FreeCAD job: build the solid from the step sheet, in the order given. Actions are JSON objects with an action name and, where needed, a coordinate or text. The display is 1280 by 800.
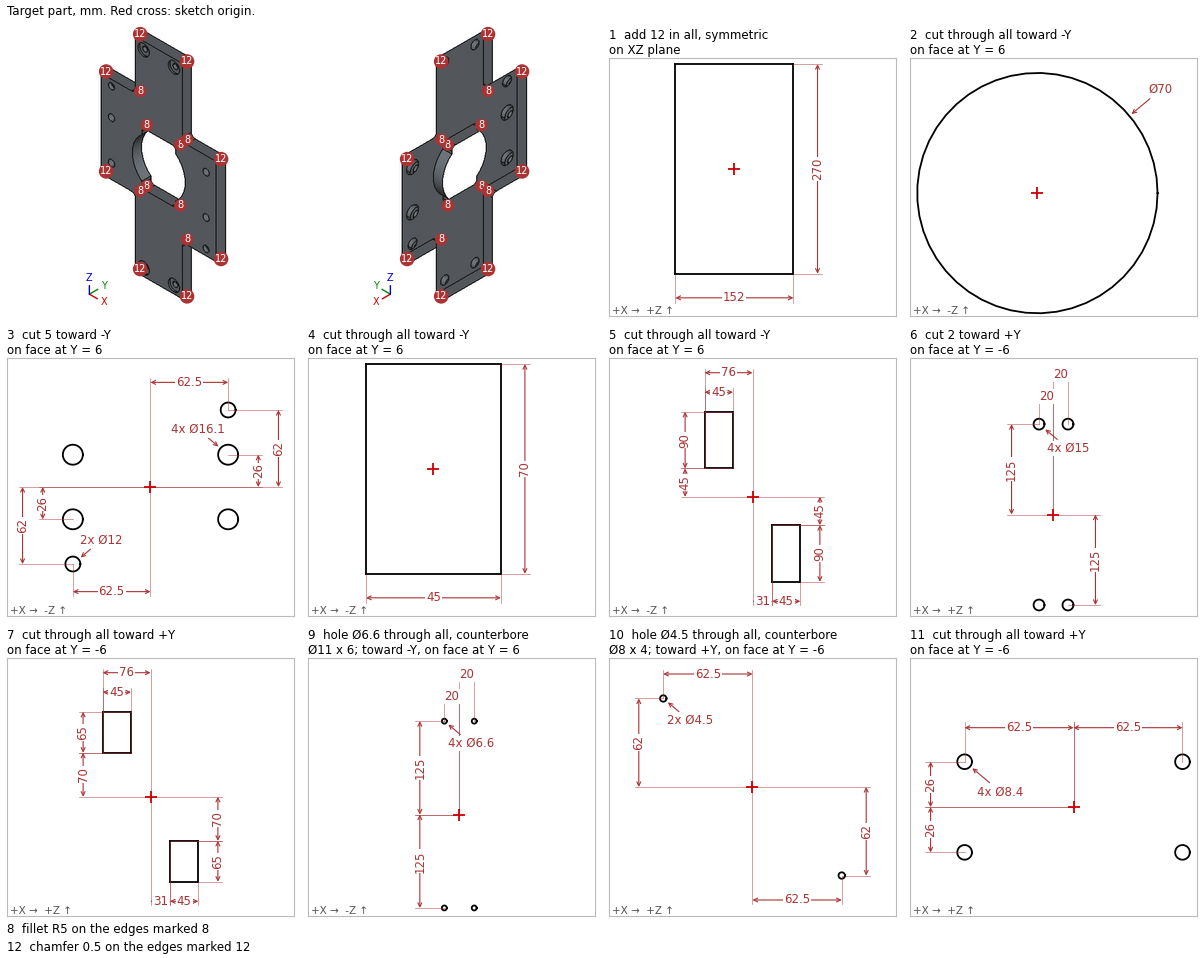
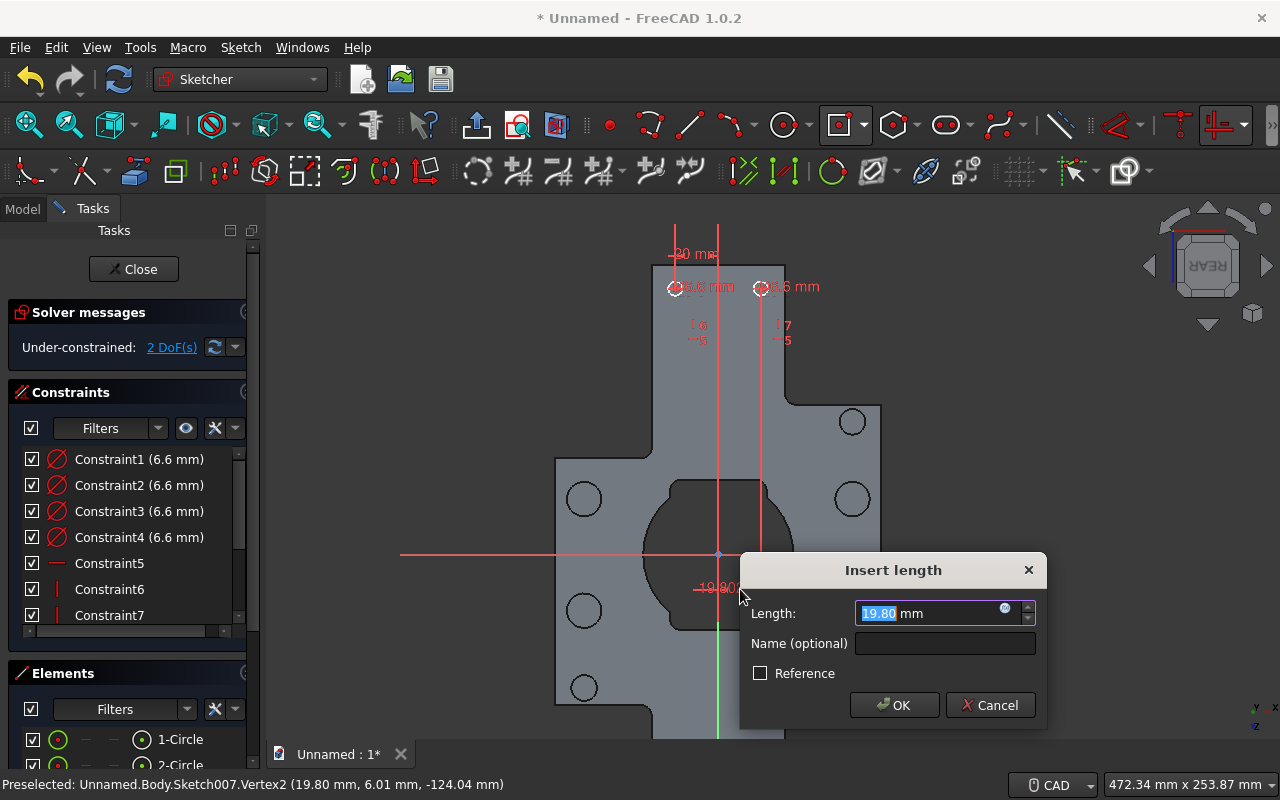
{"action": "type", "text": "20"}
{"action": "key", "text": "Return"}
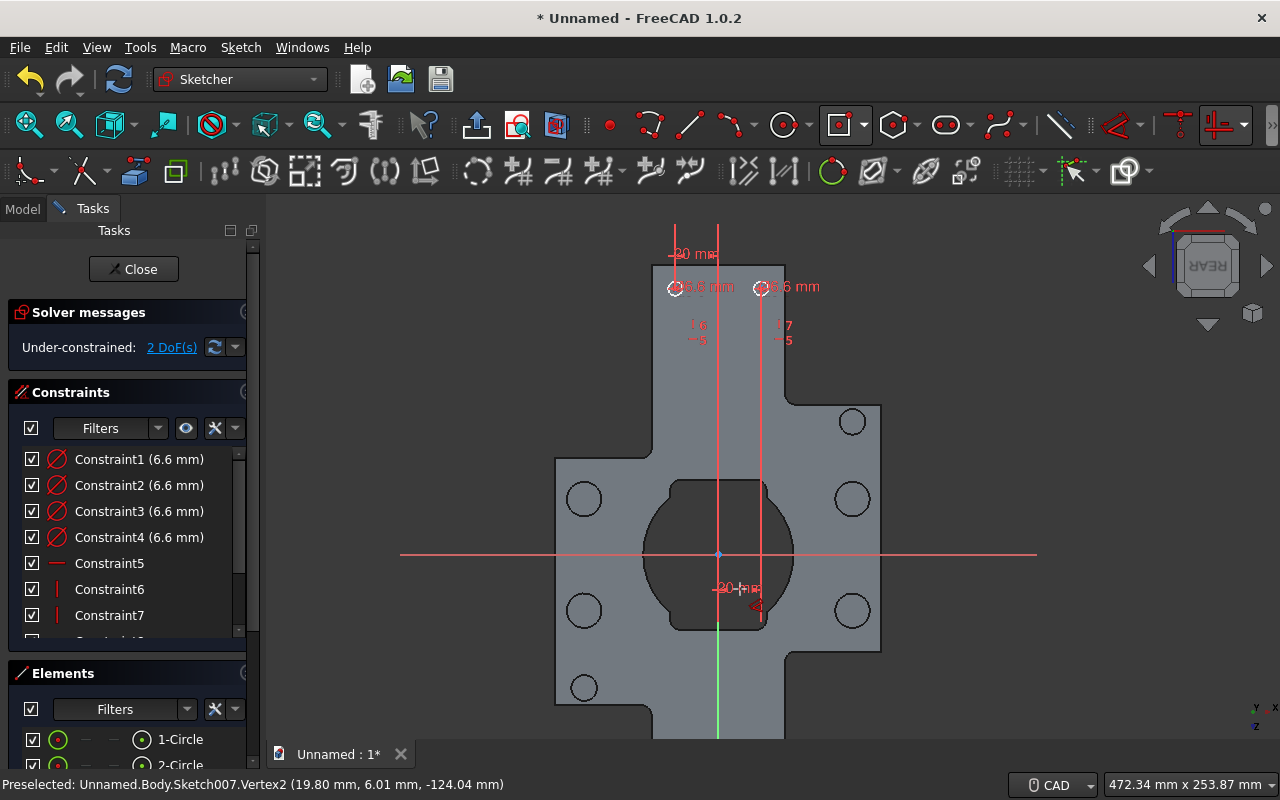
{"action": "left_click", "coordinate": [675, 289]}
{"action": "left_click", "coordinate": [641, 422]}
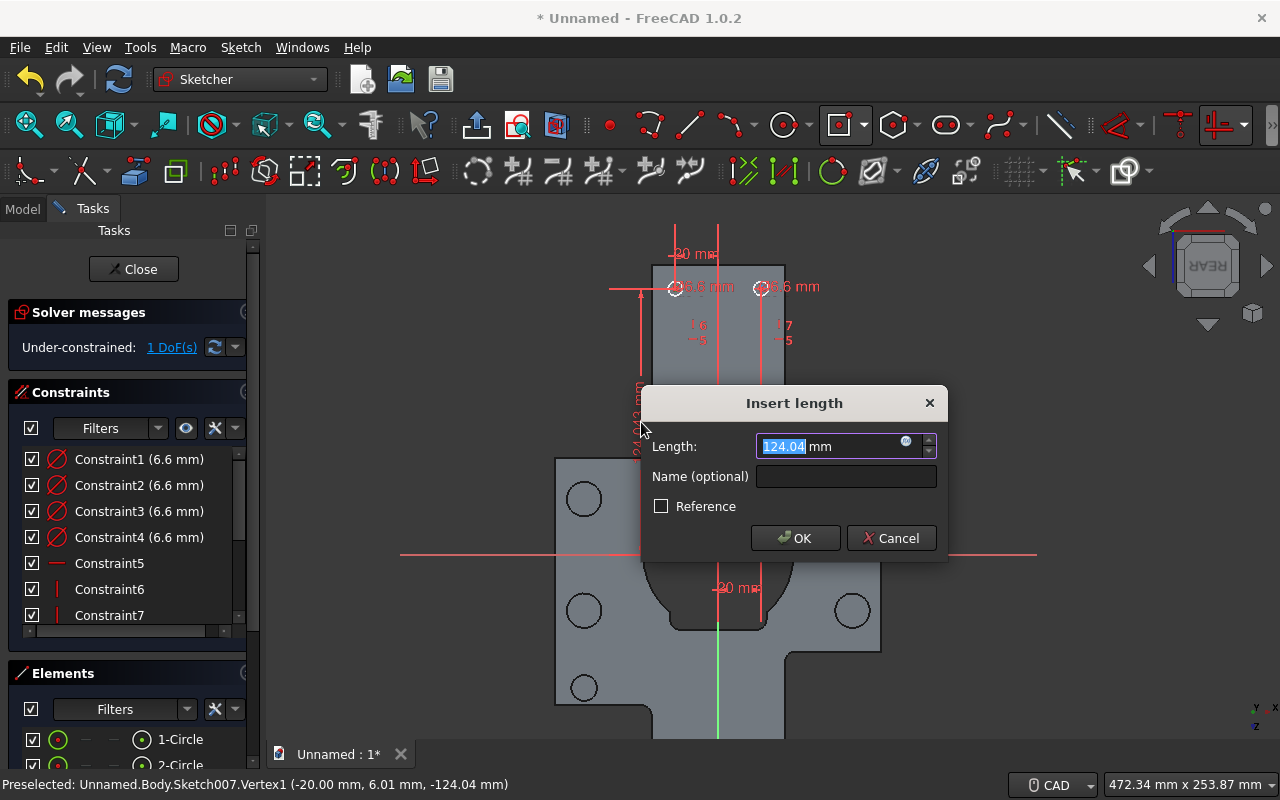
{"action": "type", "text": "125"}
{"action": "key", "text": "Return"}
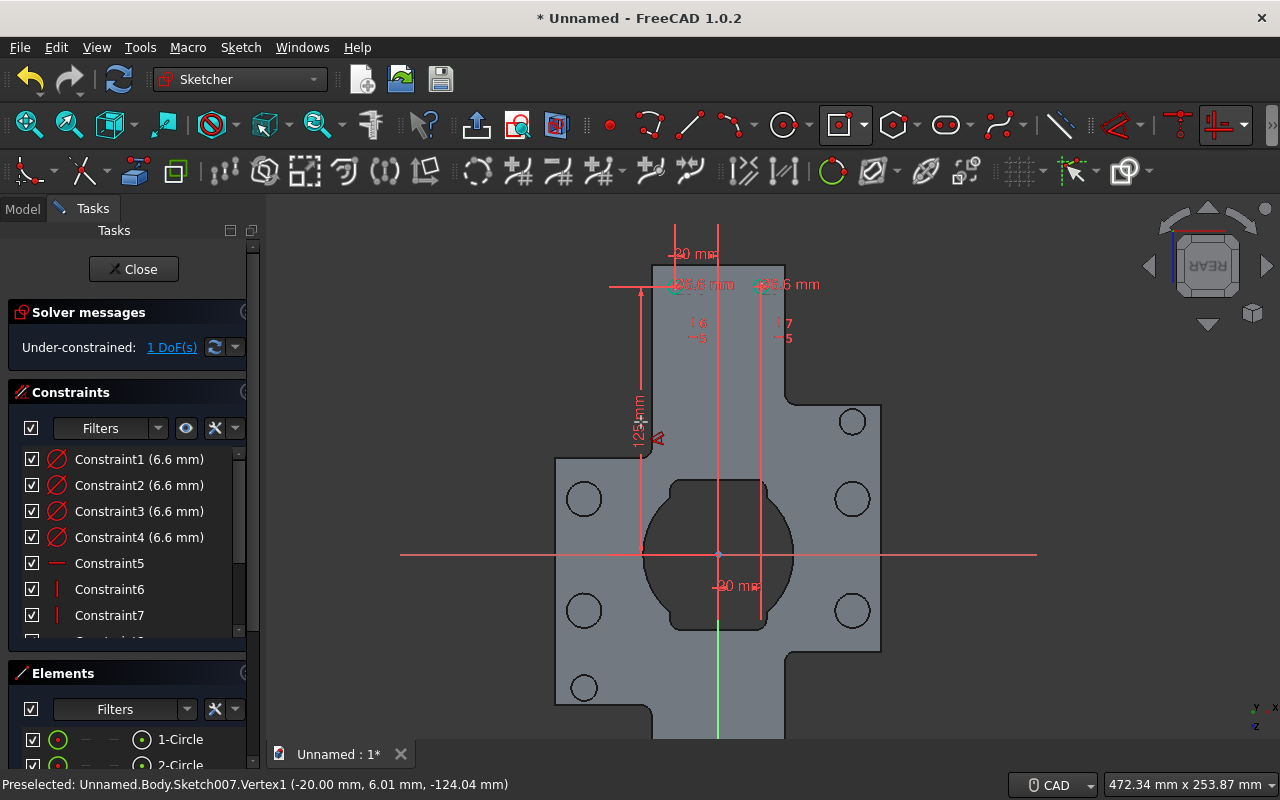
{"action": "scroll", "coordinate": [676, 287], "scroll_direction": "down", "scroll_amount": 2}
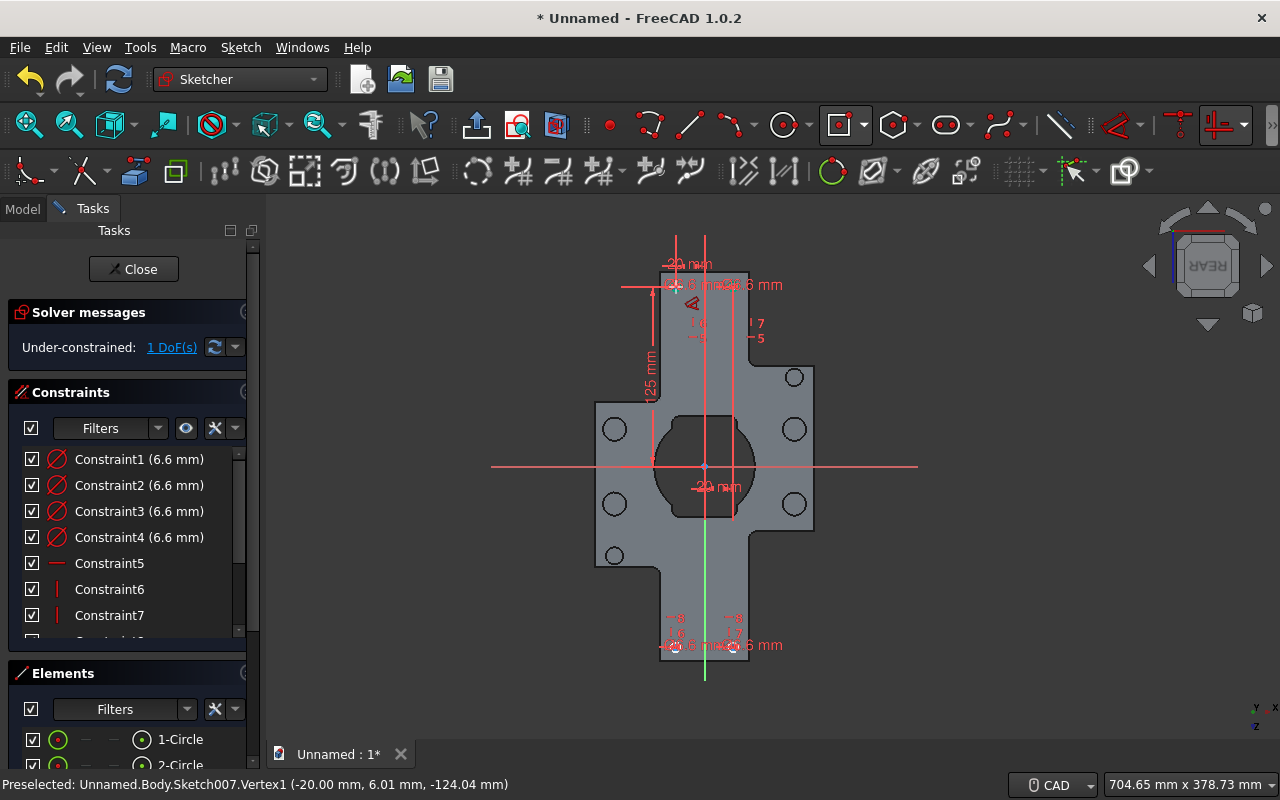
{"action": "left_click", "coordinate": [676, 647]}
{"action": "left_click", "coordinate": [642, 557]}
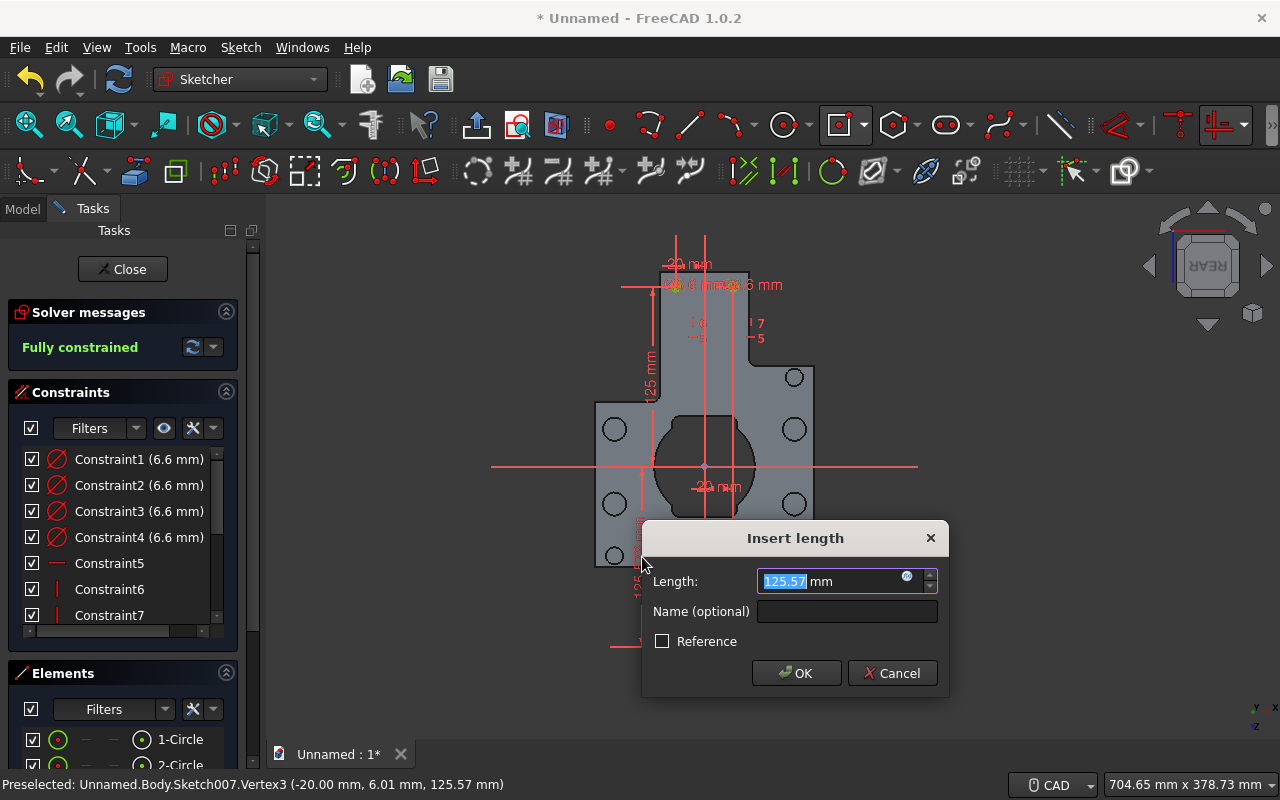
{"action": "type", "text": "125"}
{"action": "key", "text": "Return"}
{"action": "key", "text": "Escape"}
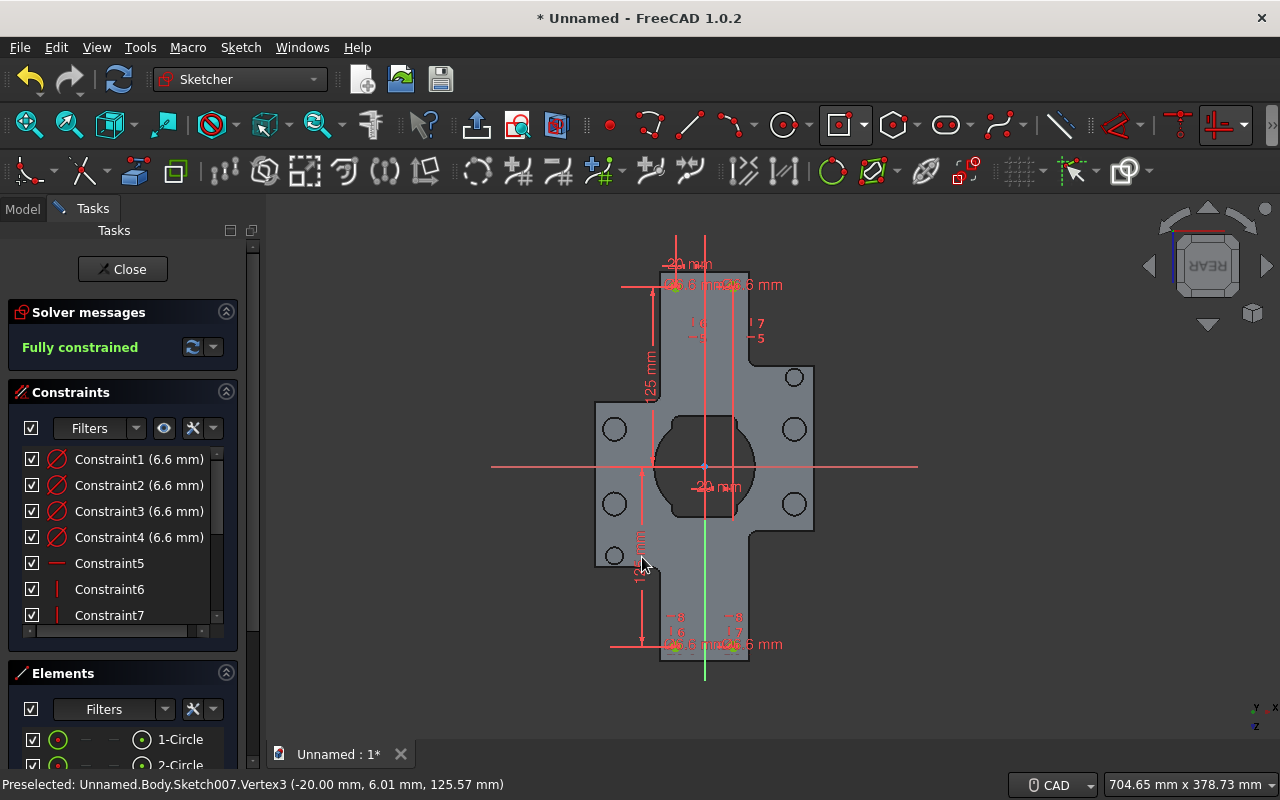
{"action": "left_click", "coordinate": [123, 269]}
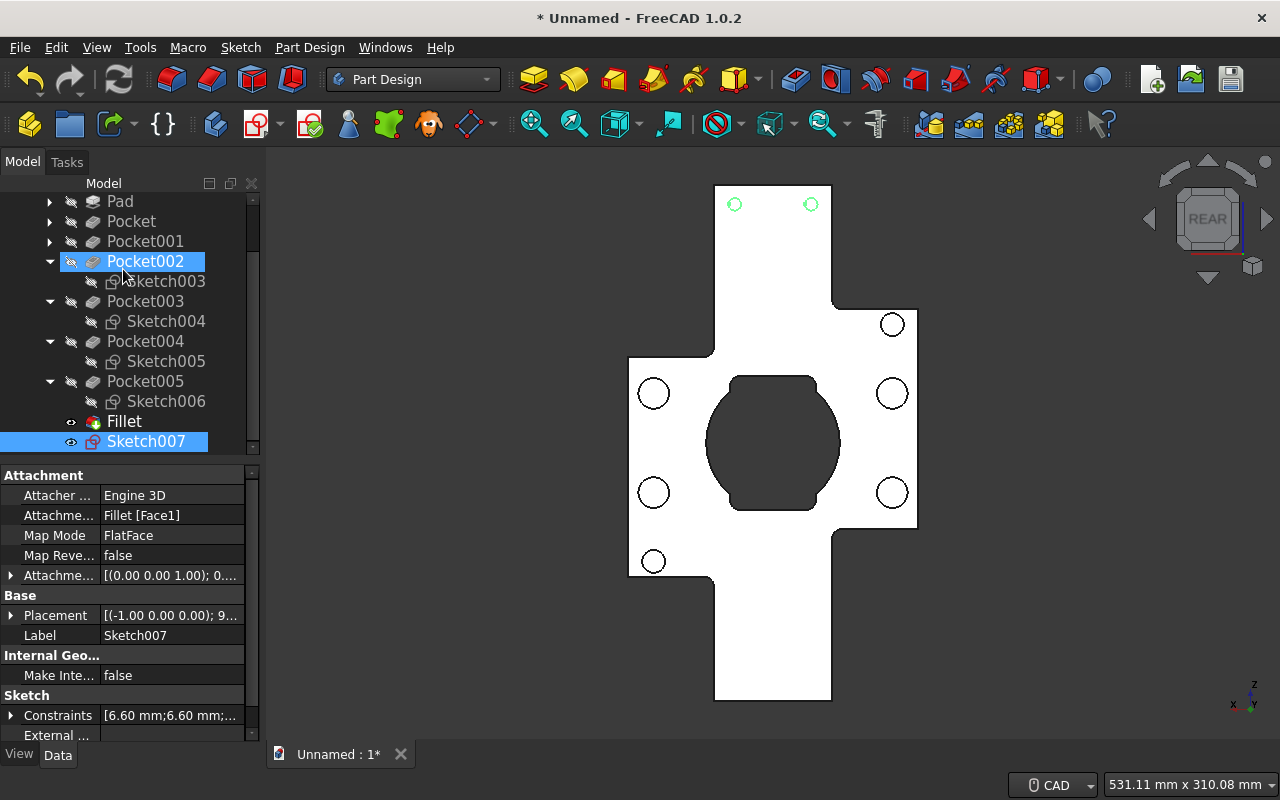
{"action": "left_click", "coordinate": [836, 80]}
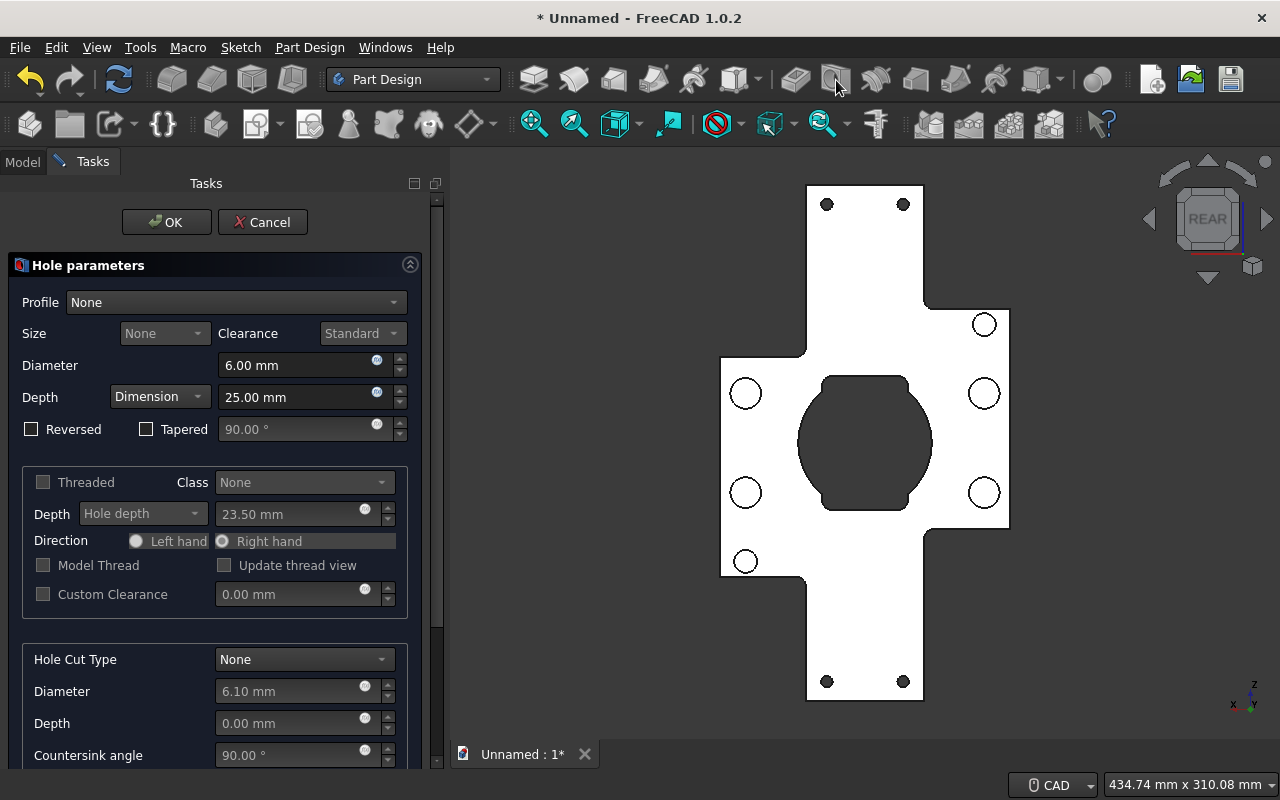
{"action": "triple_click", "coordinate": [305, 365]}